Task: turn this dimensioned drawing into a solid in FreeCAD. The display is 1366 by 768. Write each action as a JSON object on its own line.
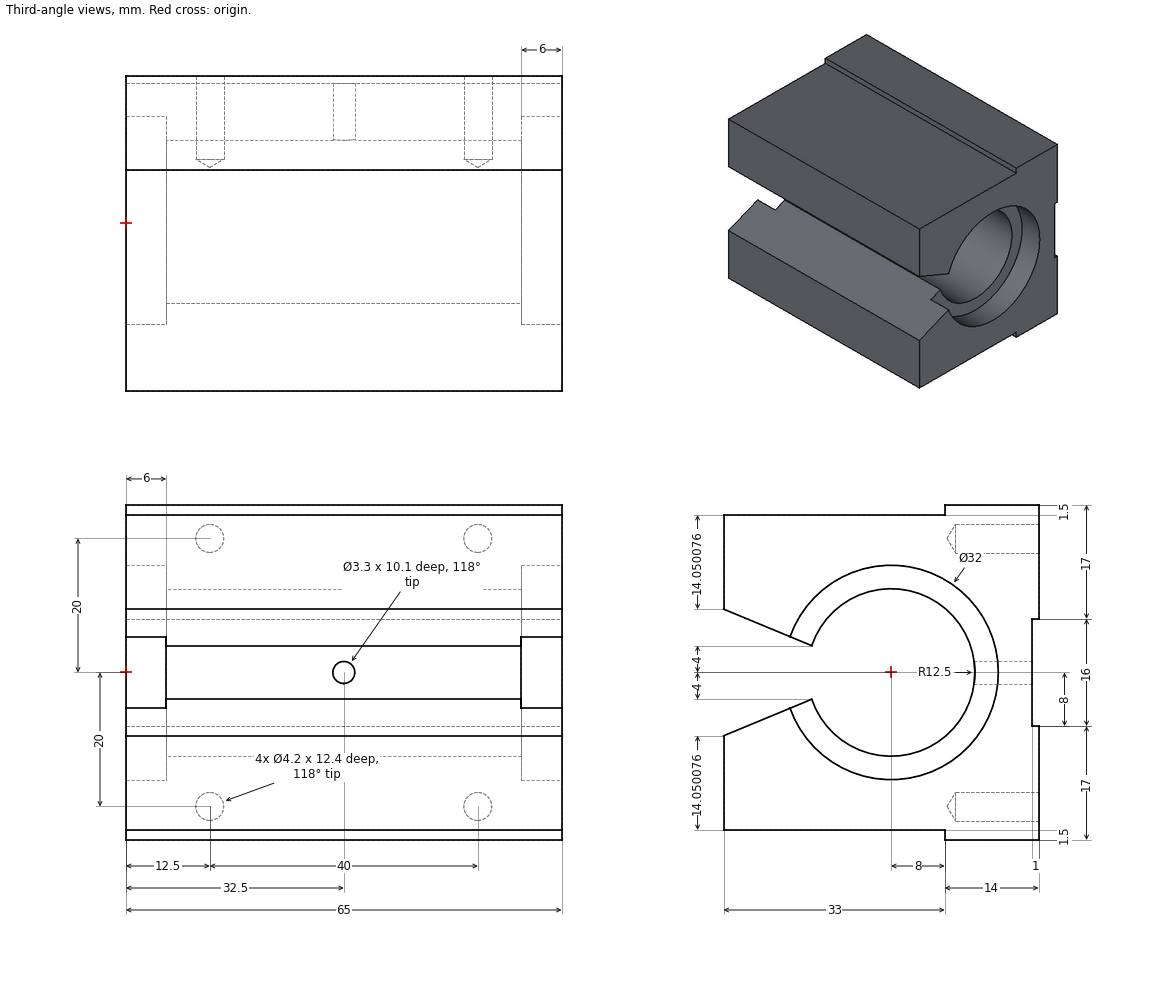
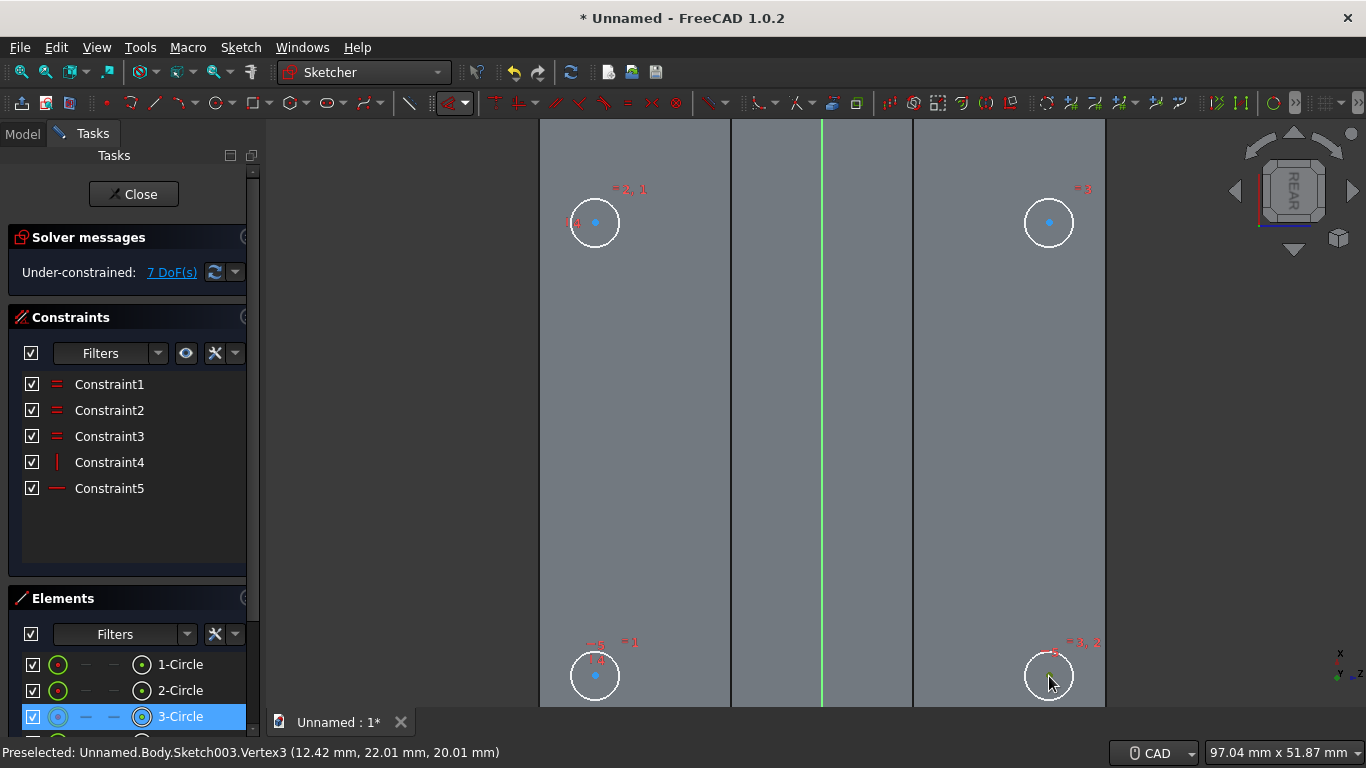
{"action": "left_click", "coordinate": [1049, 223]}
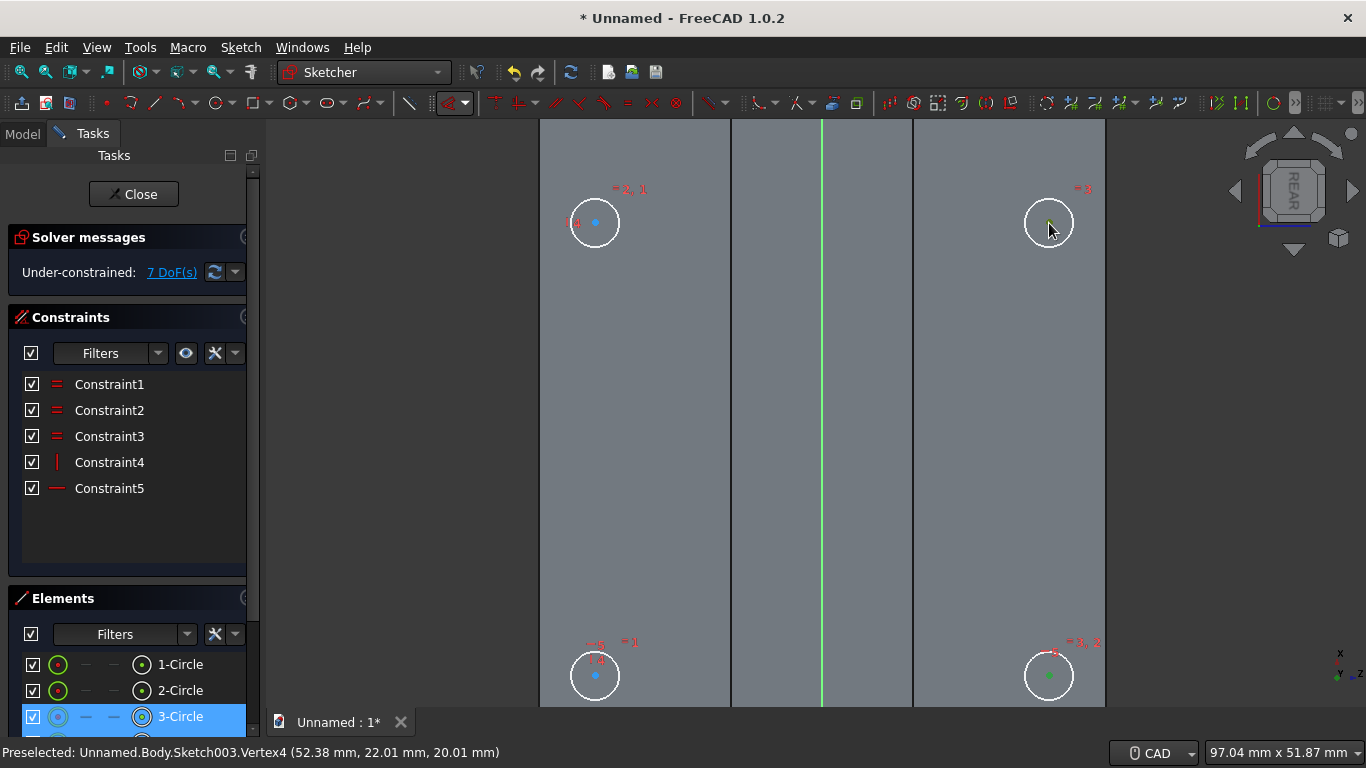
{"action": "key", "text": "v"}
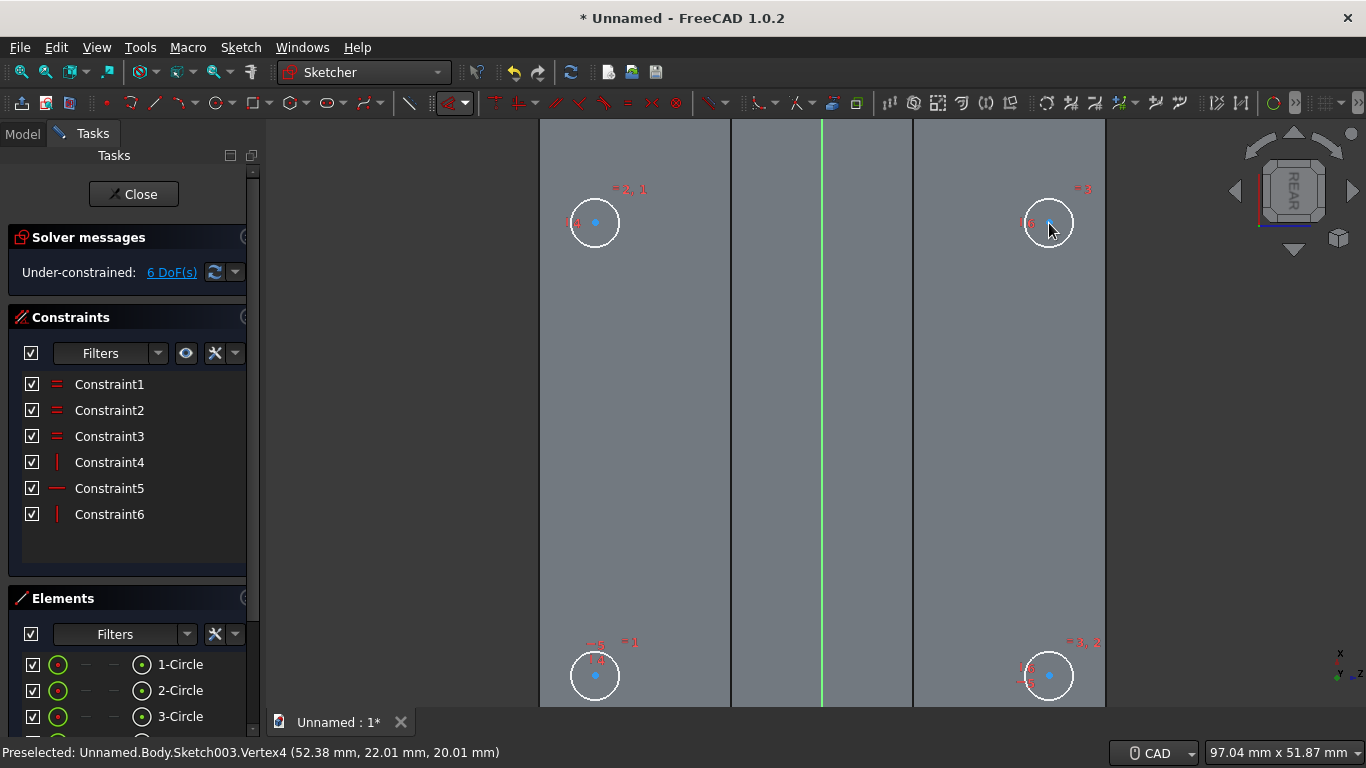
{"action": "left_click", "coordinate": [595, 223]}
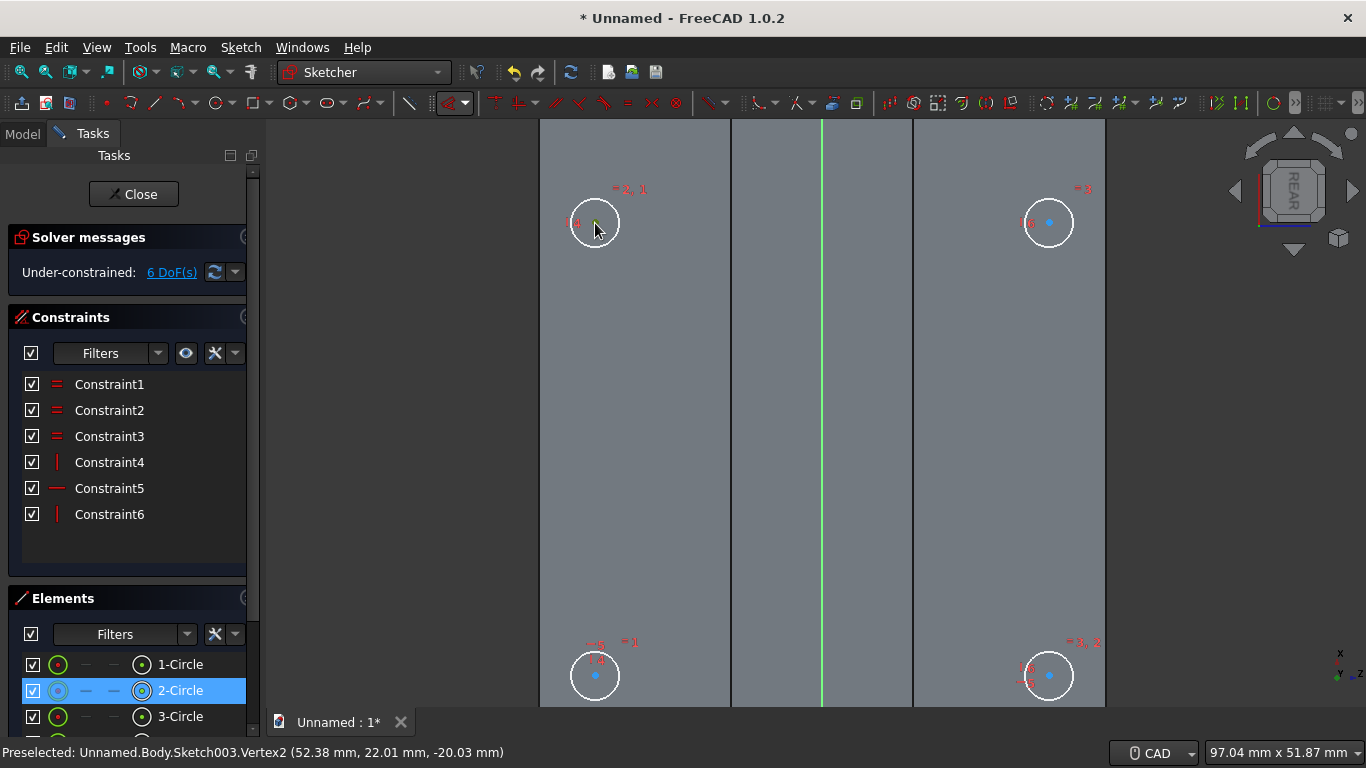
{"action": "left_click", "coordinate": [1049, 223]}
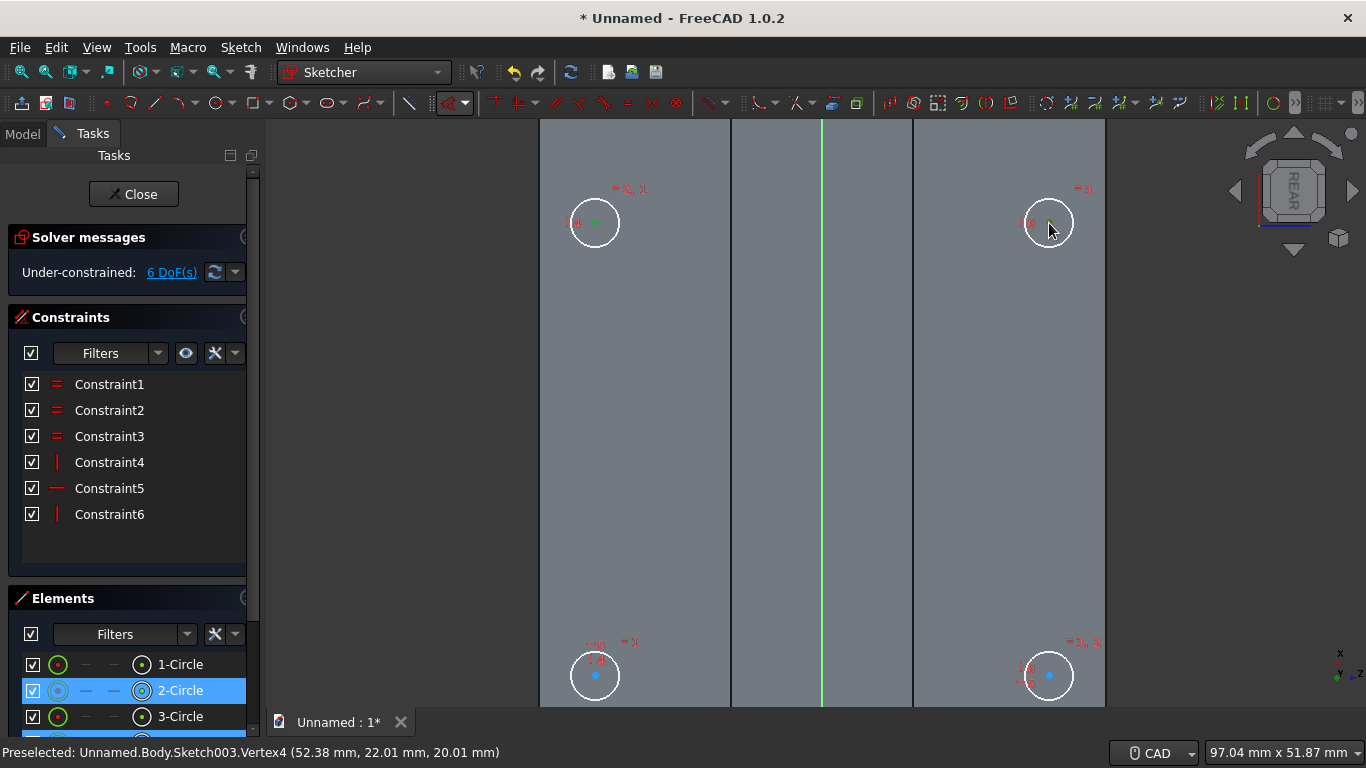
{"action": "key", "text": "h"}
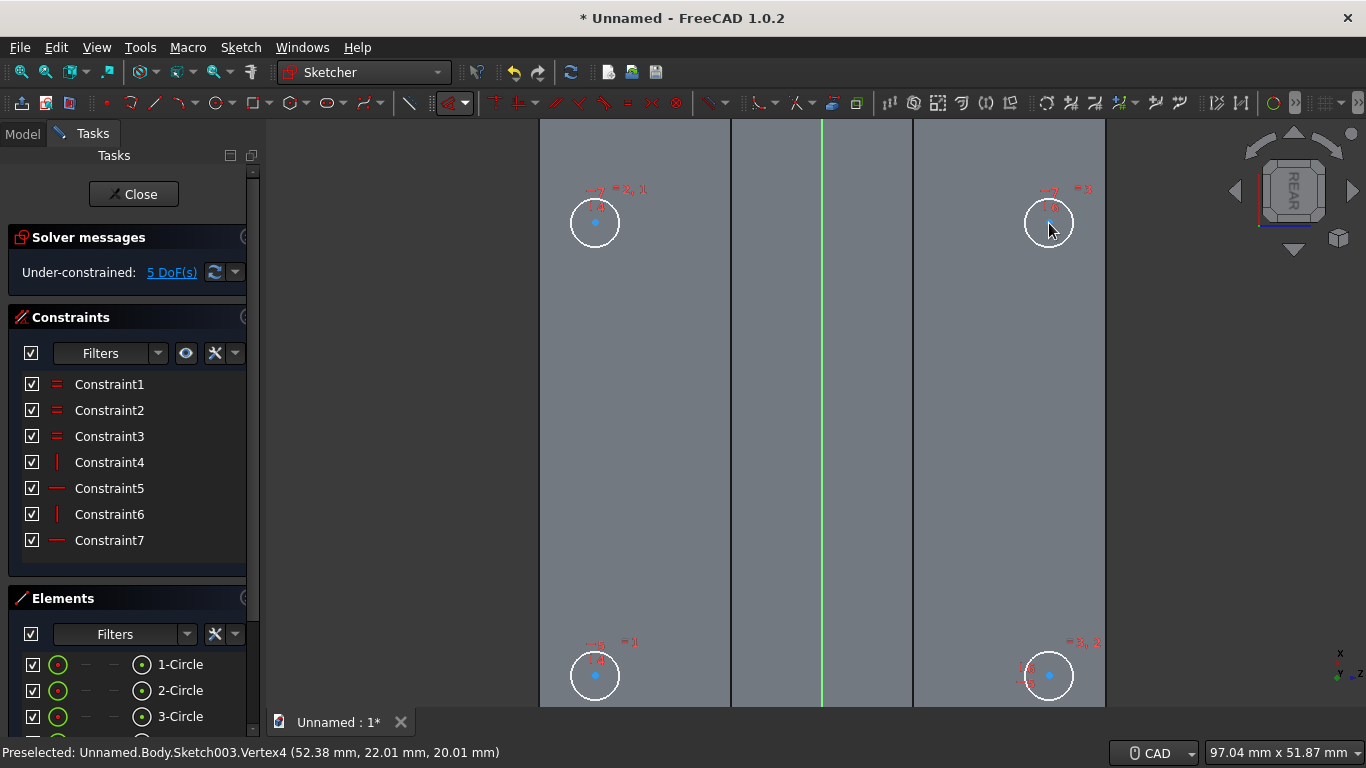
{"action": "left_click", "coordinate": [612, 659]}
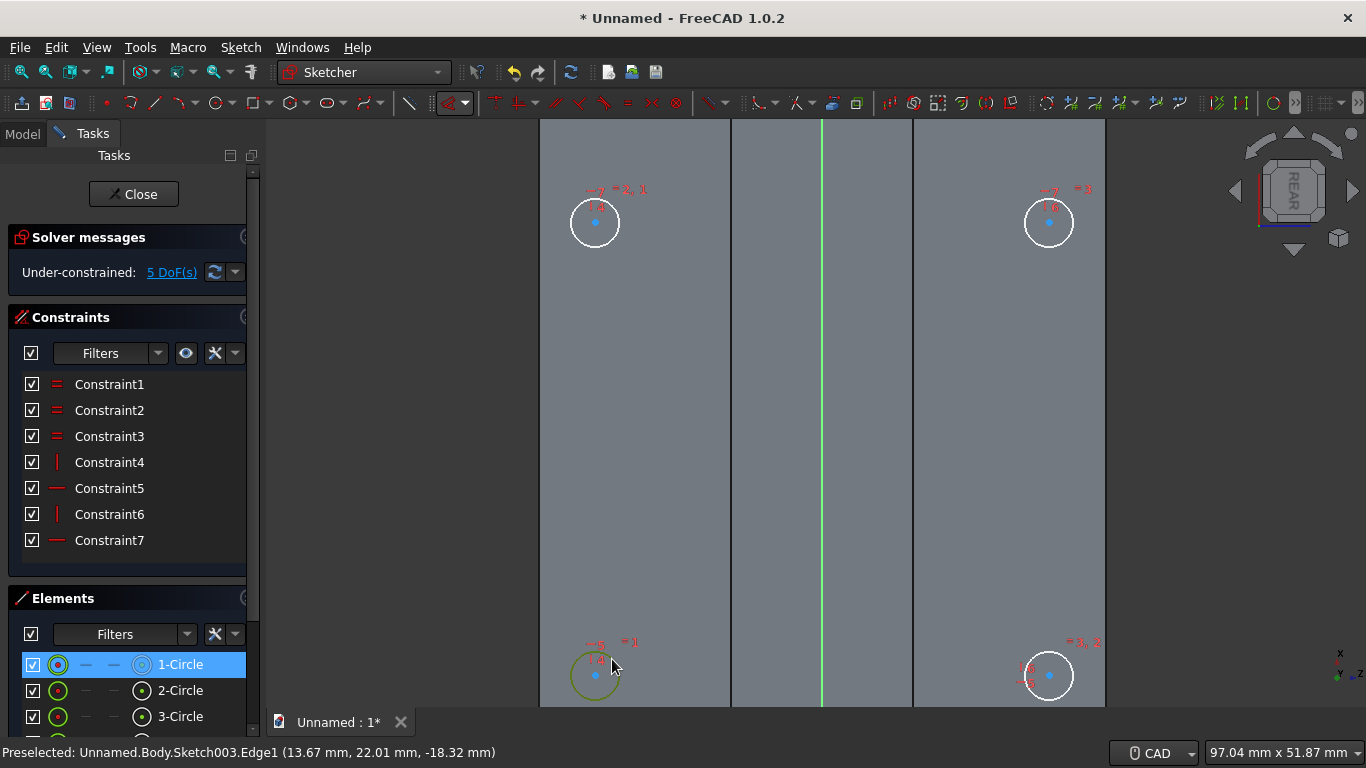
{"action": "key", "text": "k o"}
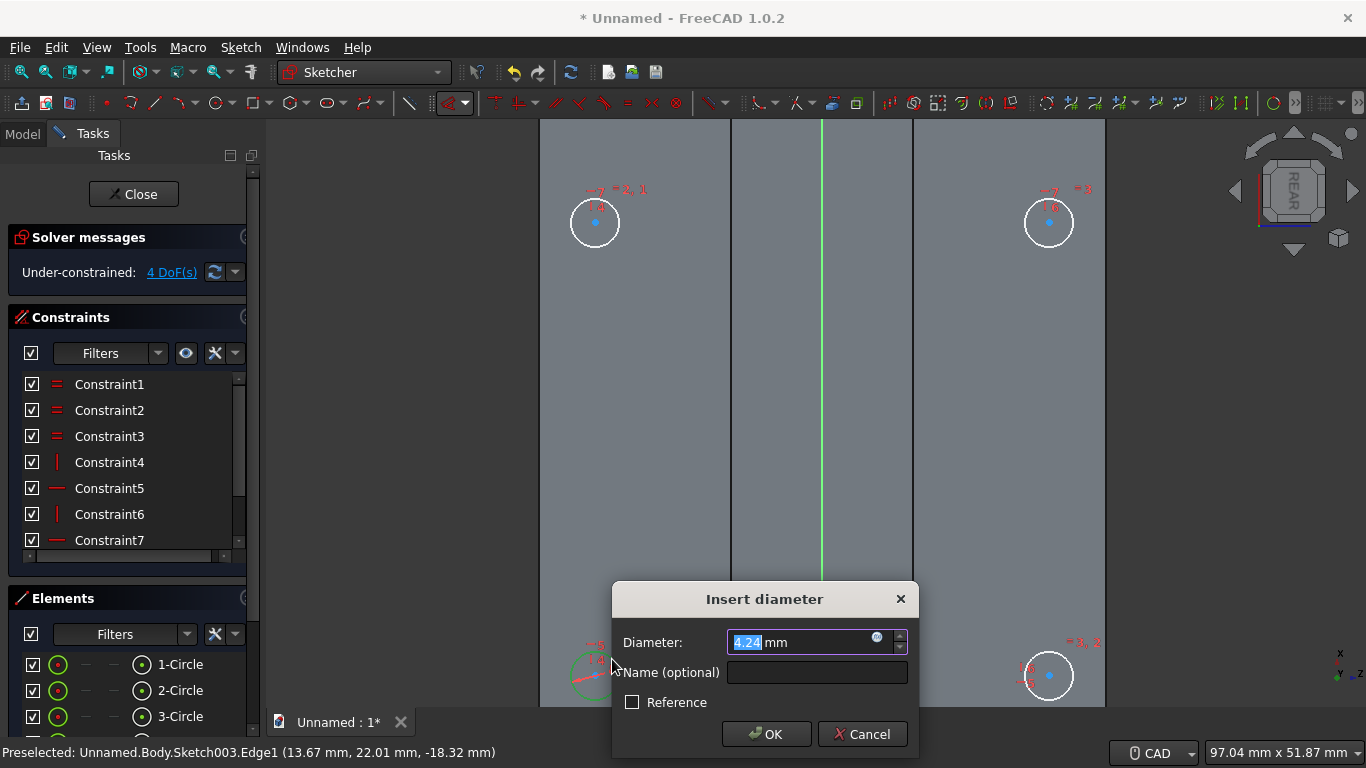
{"action": "type", "text": "4.2"}
{"action": "key", "text": "Return"}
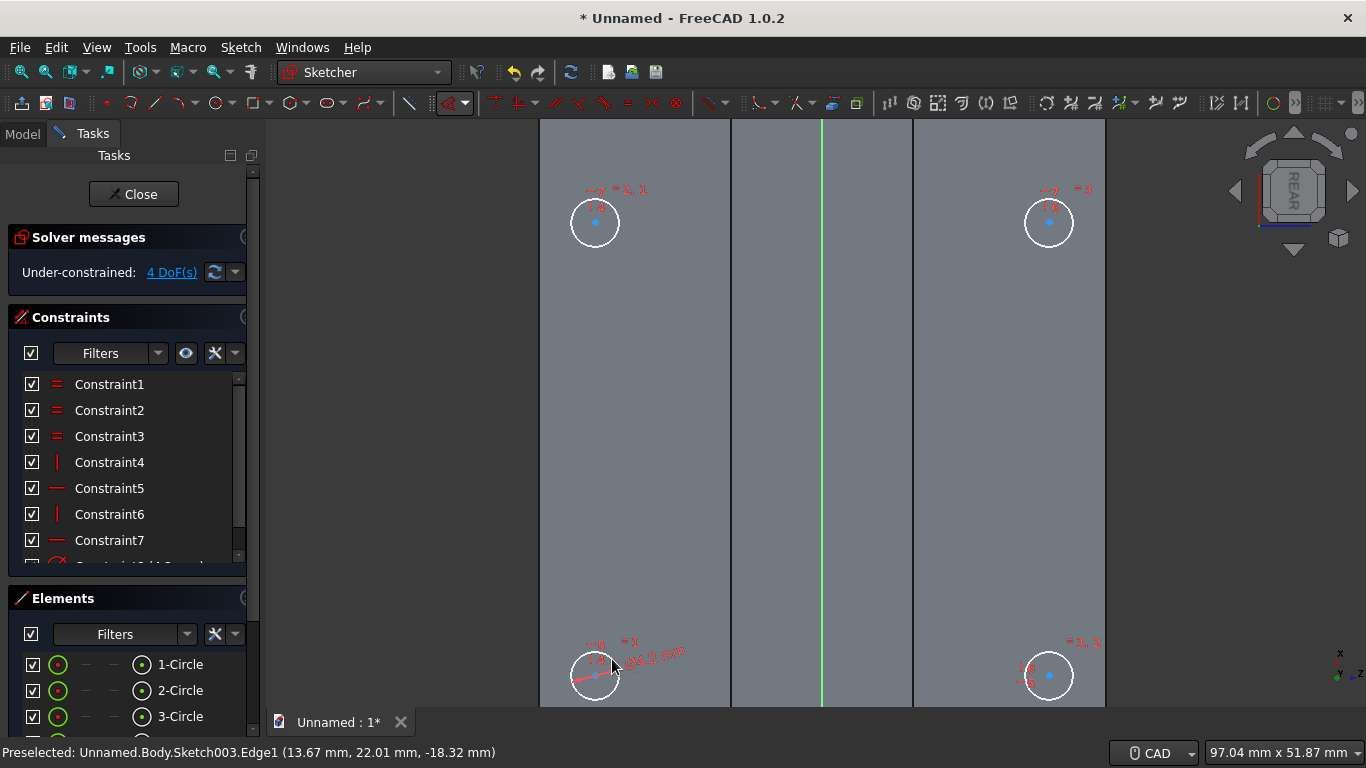
{"action": "left_click", "coordinate": [595, 676]}